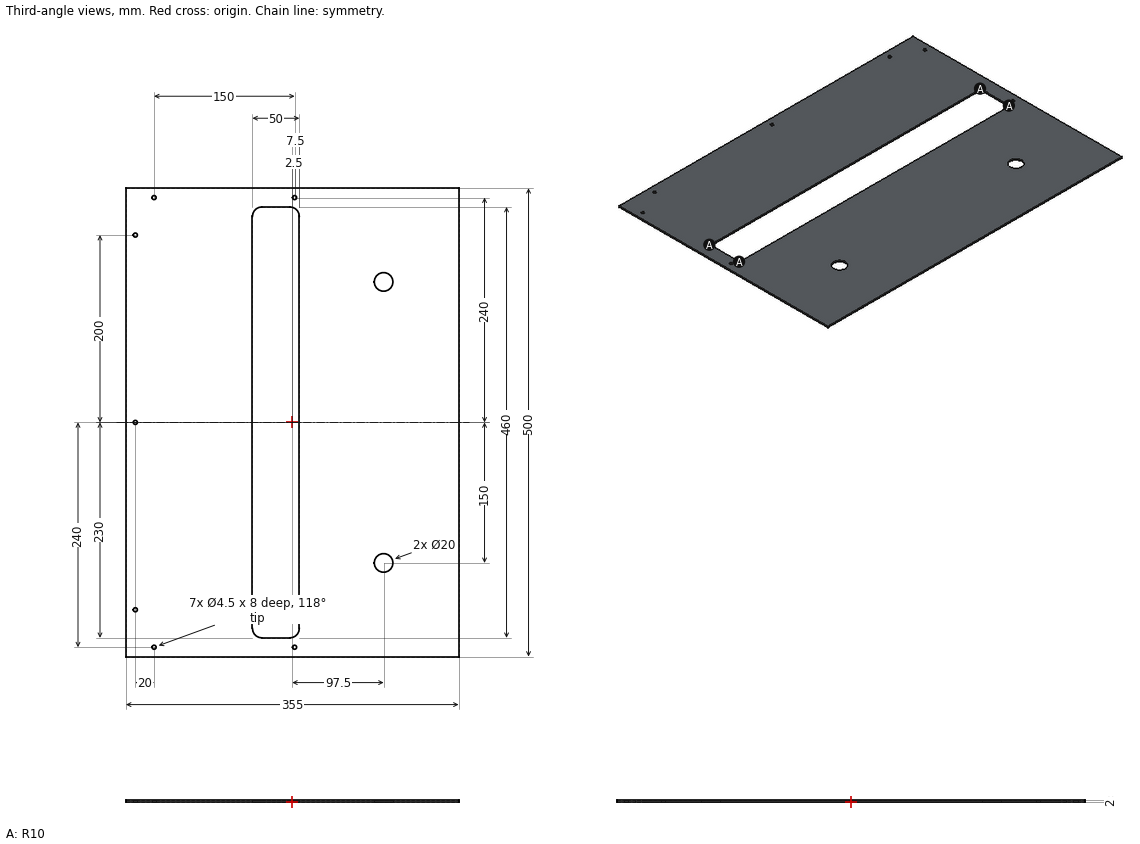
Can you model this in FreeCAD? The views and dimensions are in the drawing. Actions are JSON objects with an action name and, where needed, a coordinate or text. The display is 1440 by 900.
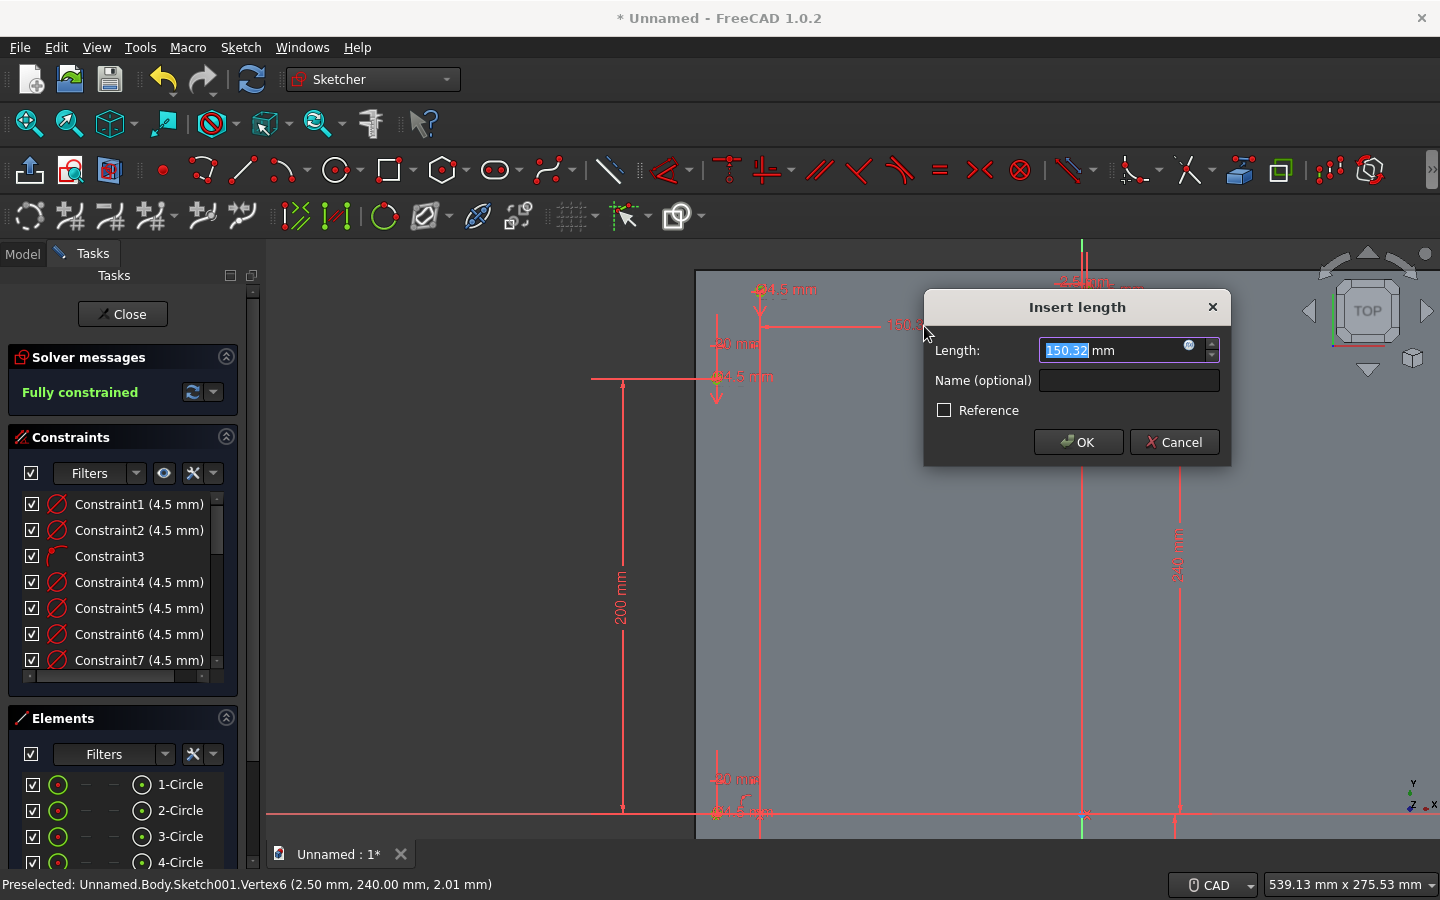
{"action": "type", "text": "150"}
{"action": "key", "text": "Return"}
{"action": "key", "text": "Escape"}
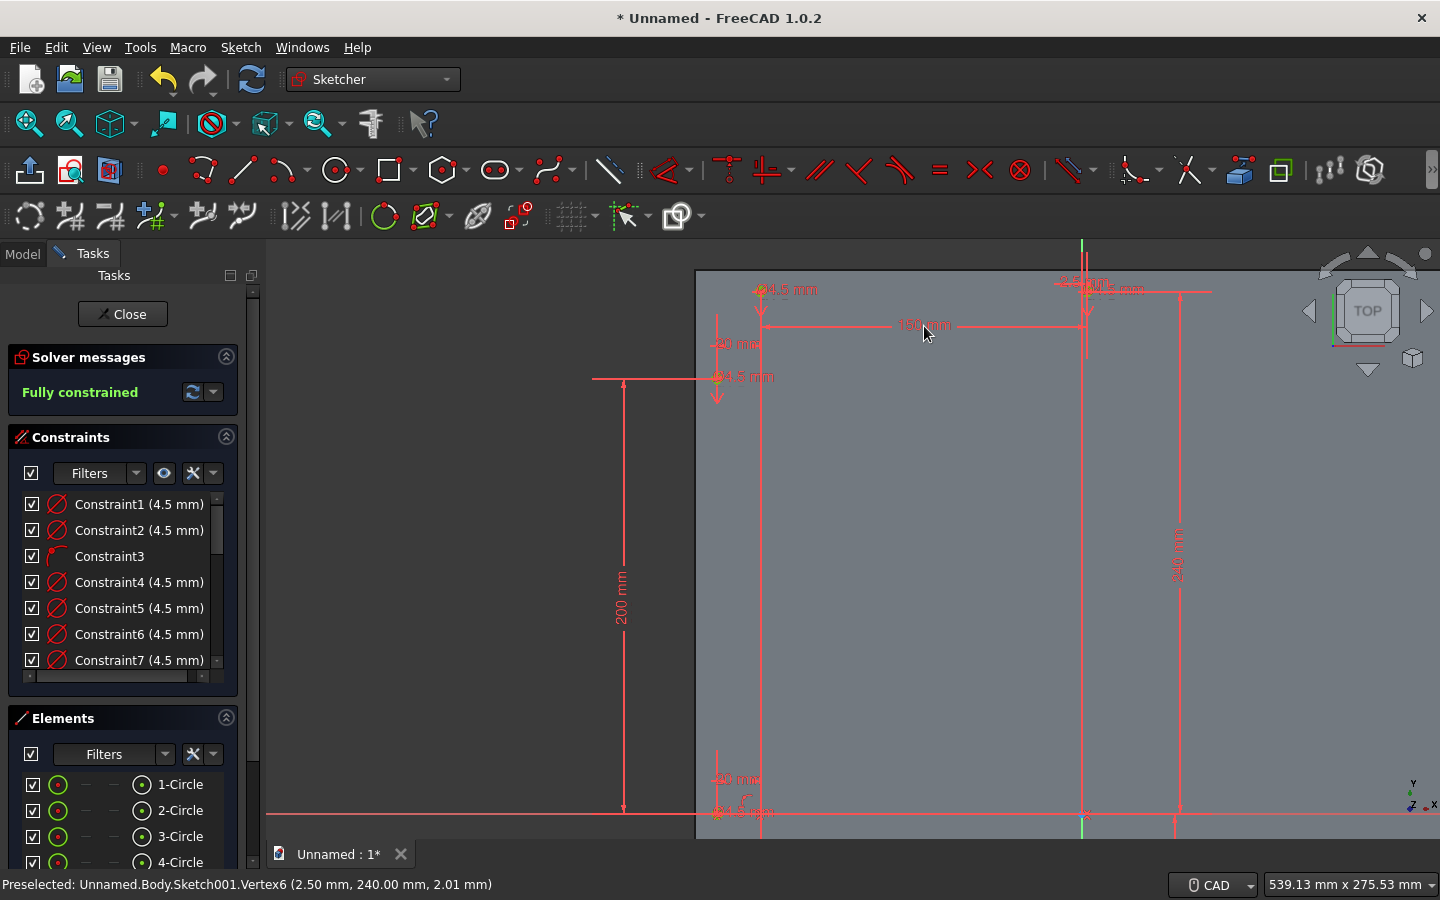
{"action": "left_click", "coordinate": [123, 314]}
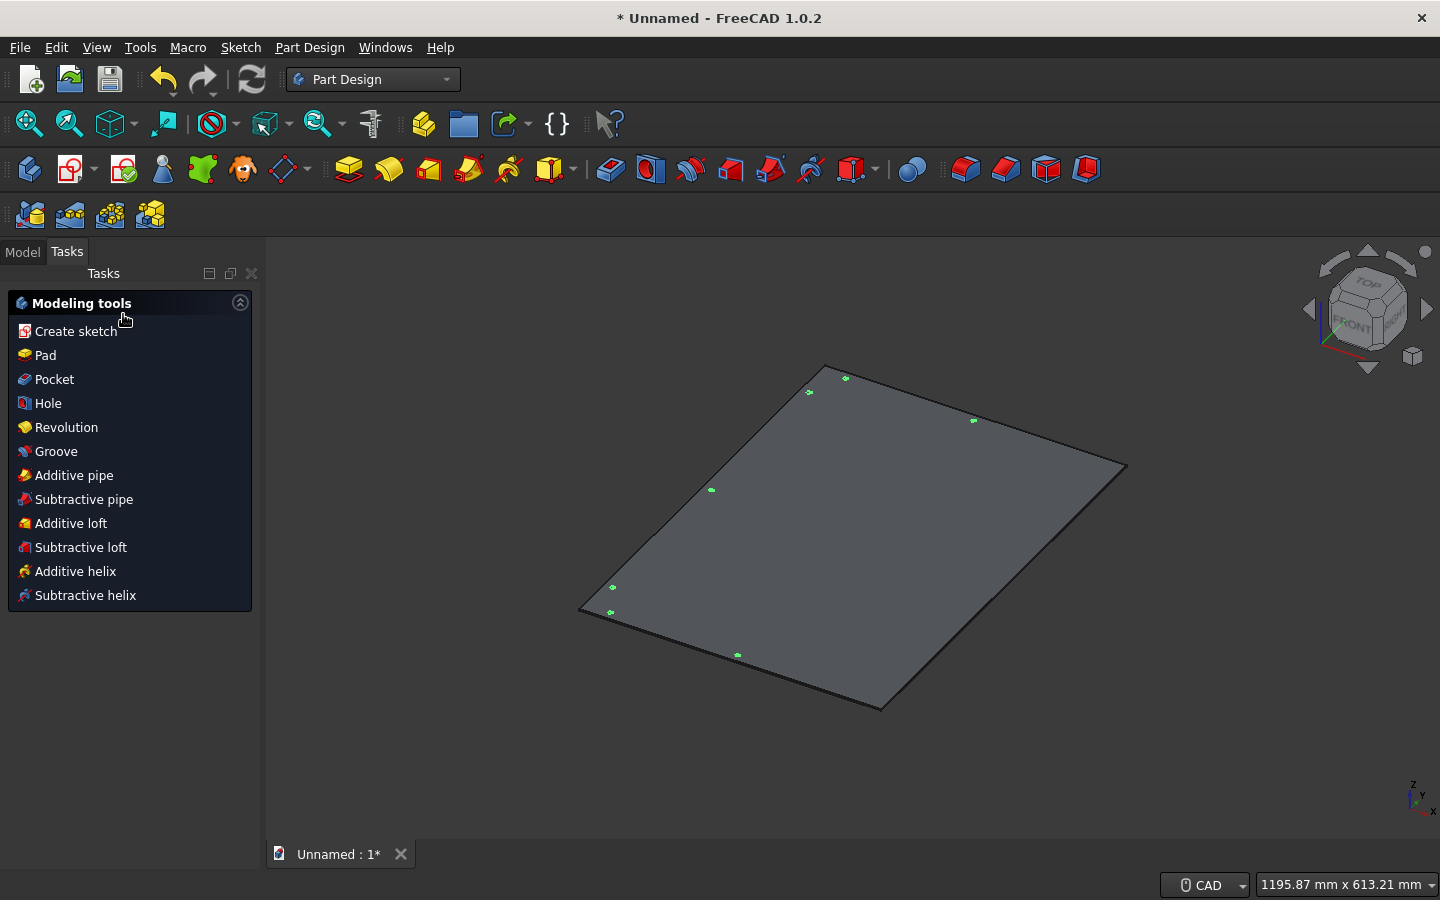
{"action": "left_click", "coordinate": [652, 170]}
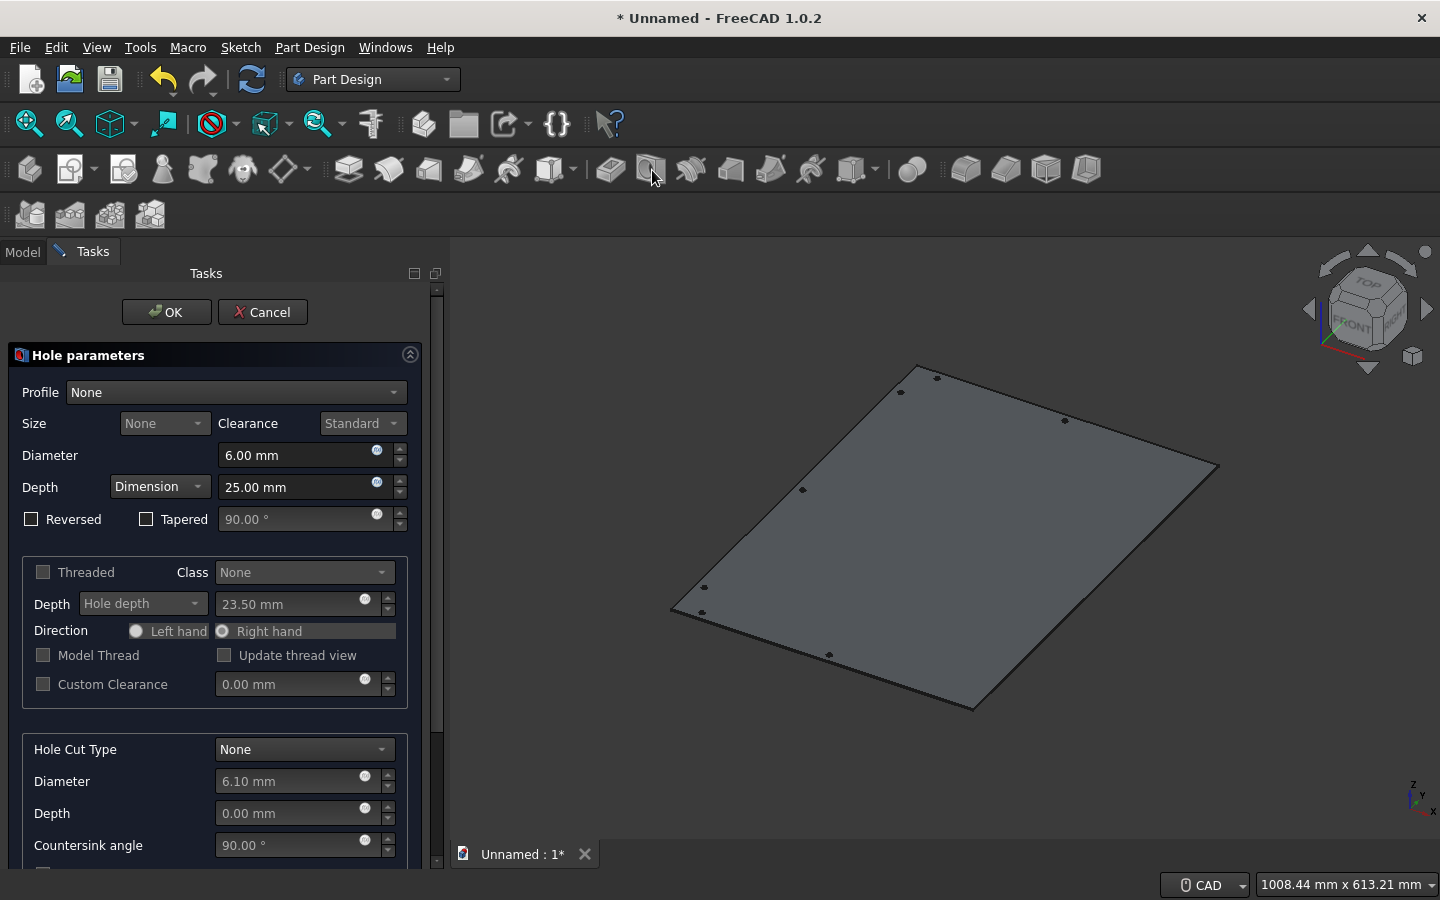
{"action": "triple_click", "coordinate": [305, 455]}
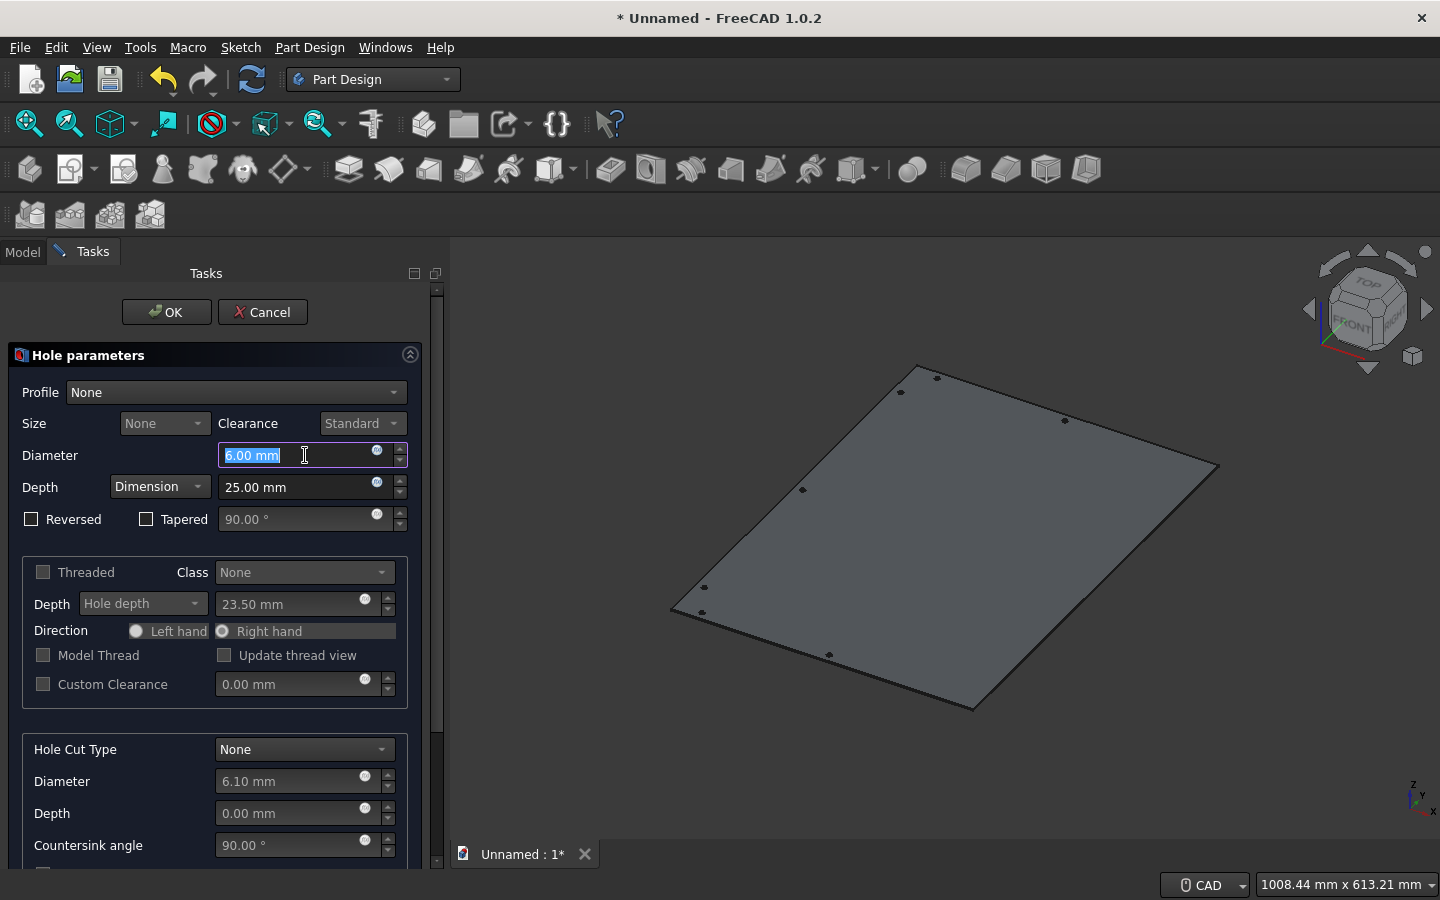
{"action": "type", "text": "4.5"}
{"action": "key", "text": "Tab"}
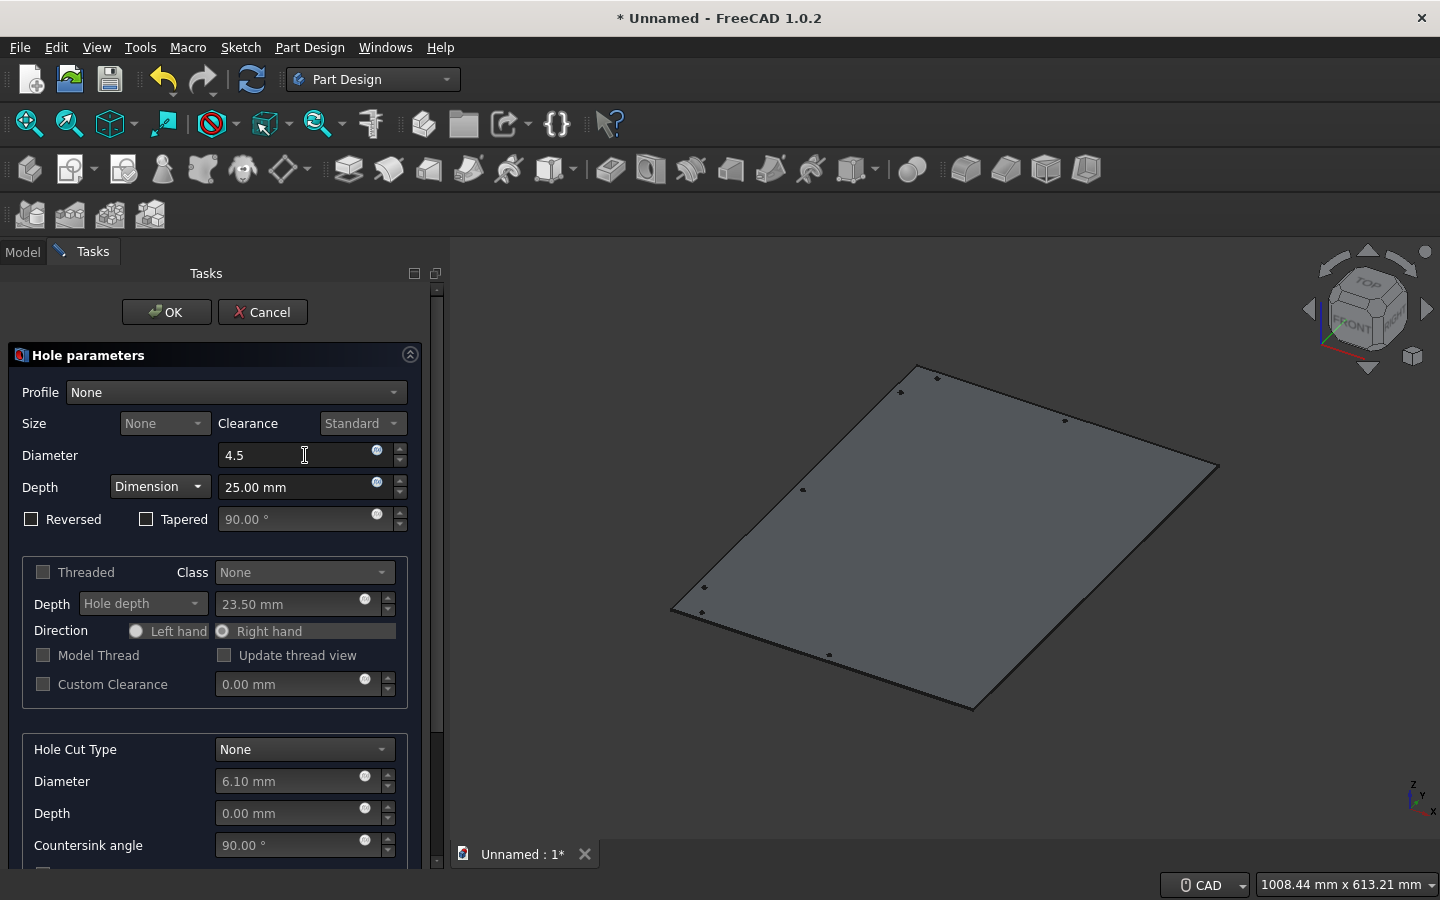
{"action": "triple_click", "coordinate": [305, 487]}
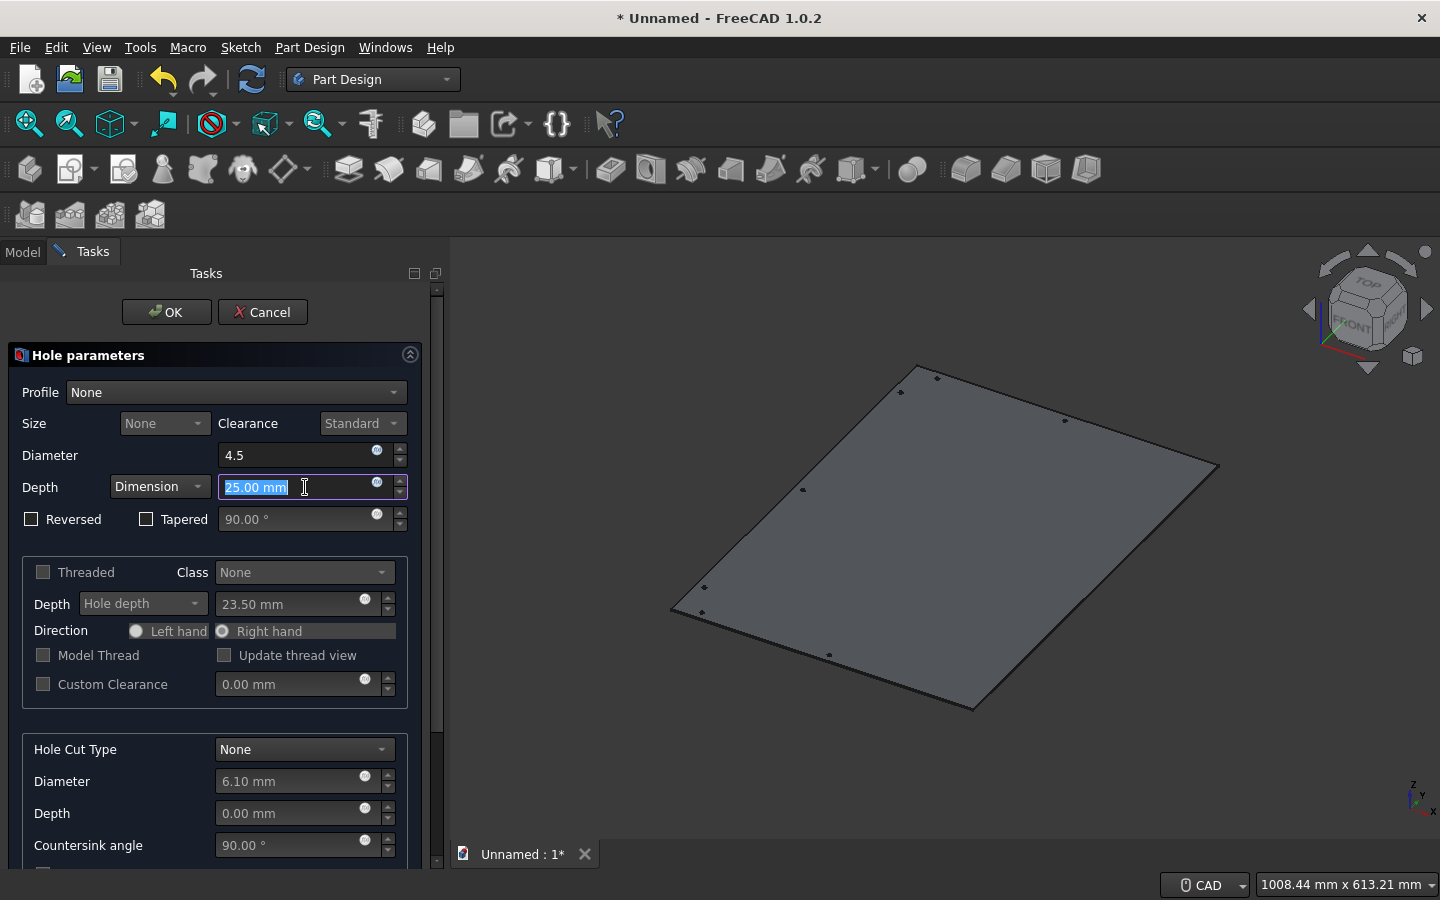
{"action": "type", "text": "8"}
{"action": "key", "text": "Tab"}